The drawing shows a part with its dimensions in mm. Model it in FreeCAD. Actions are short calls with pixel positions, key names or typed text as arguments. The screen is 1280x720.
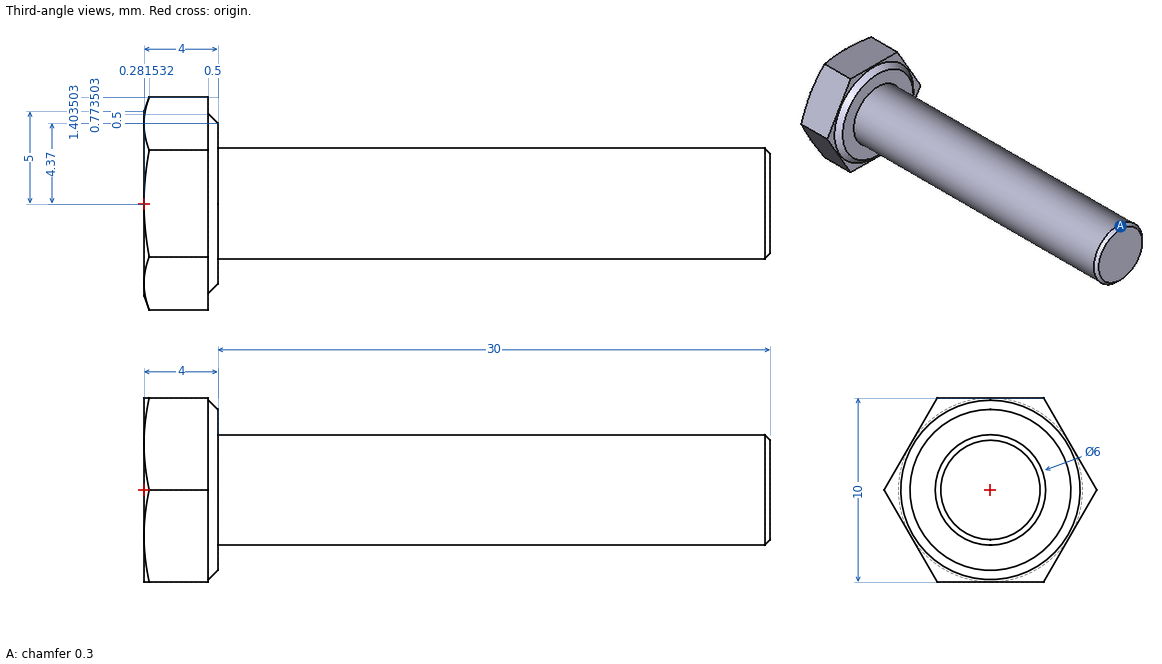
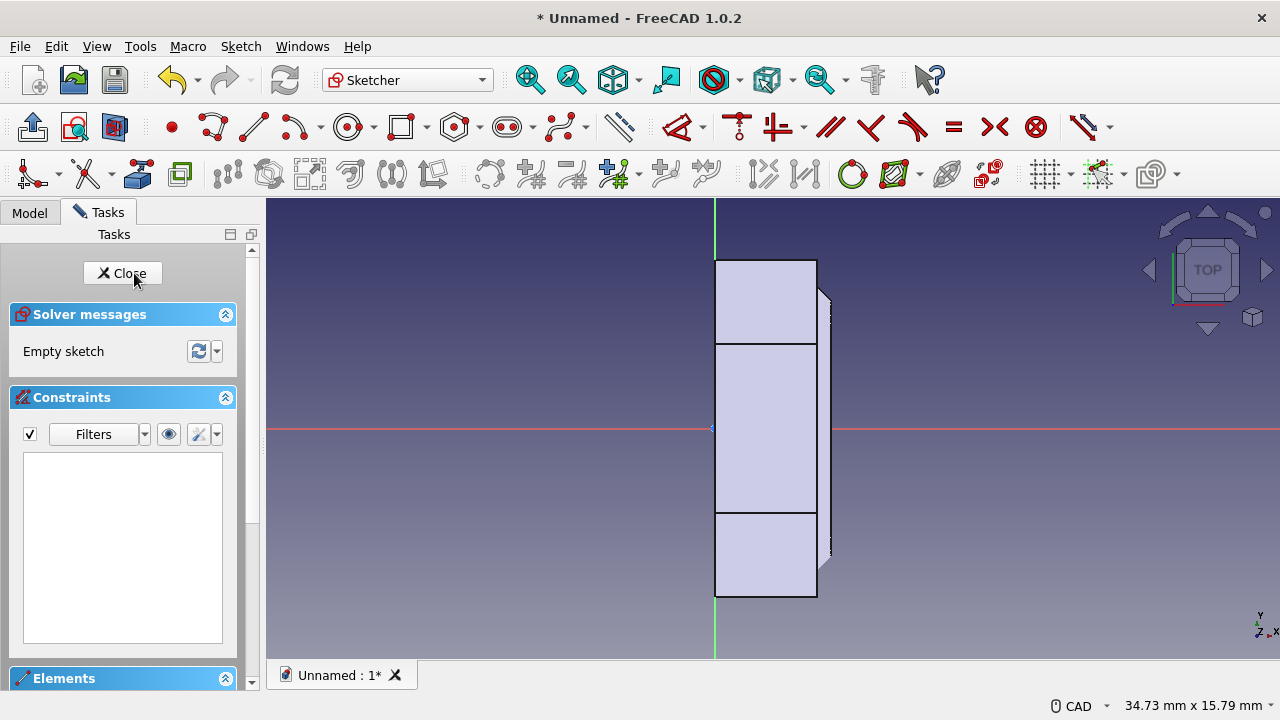
click(115, 128)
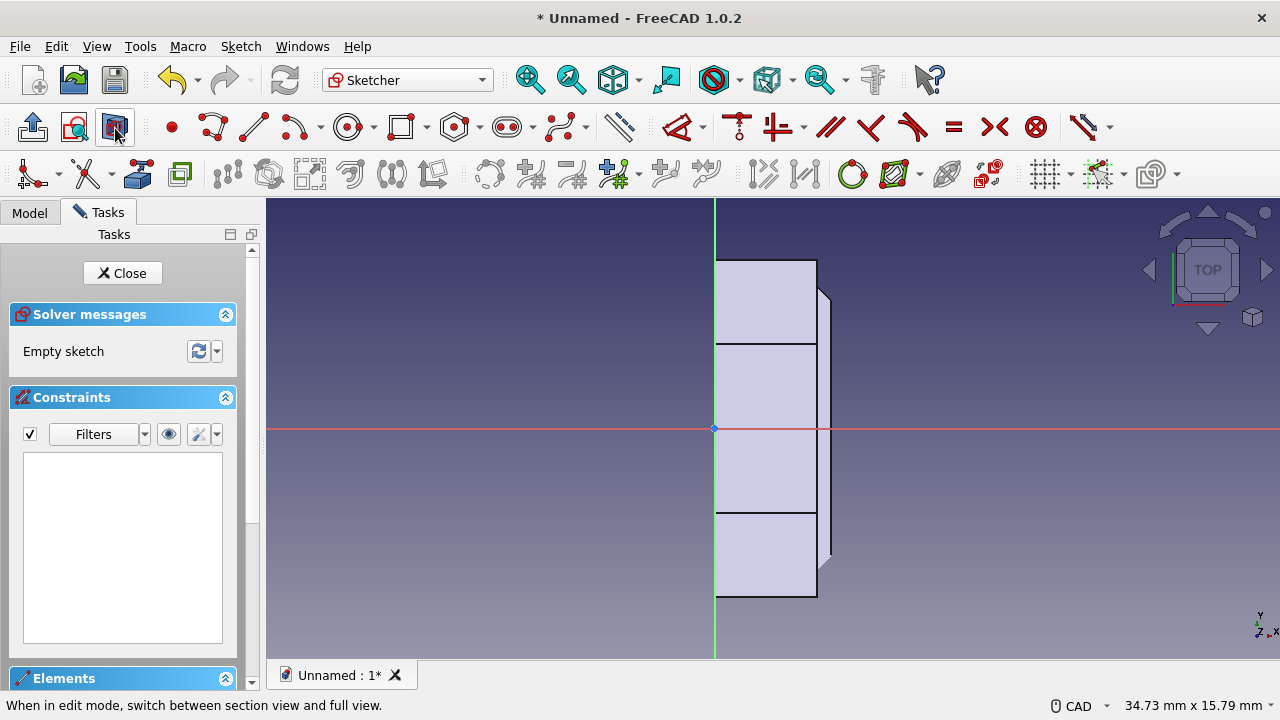
scroll(720, 259, up, 13)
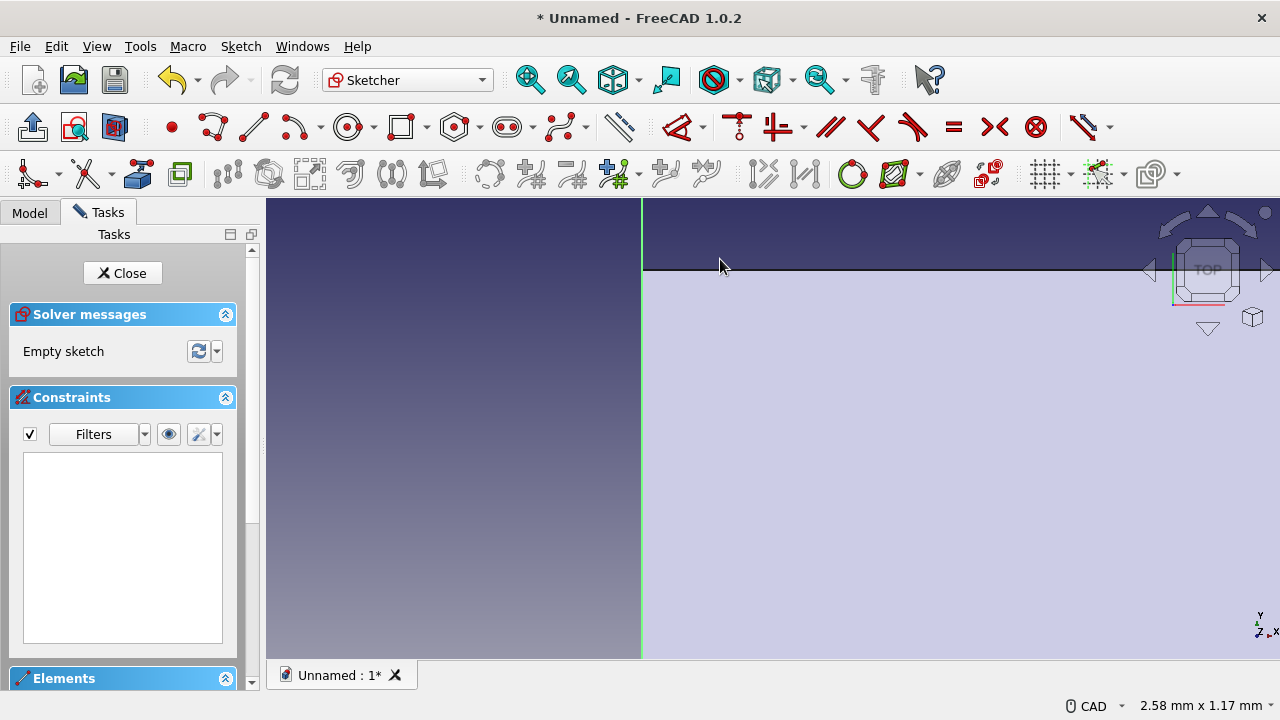
click(213, 128)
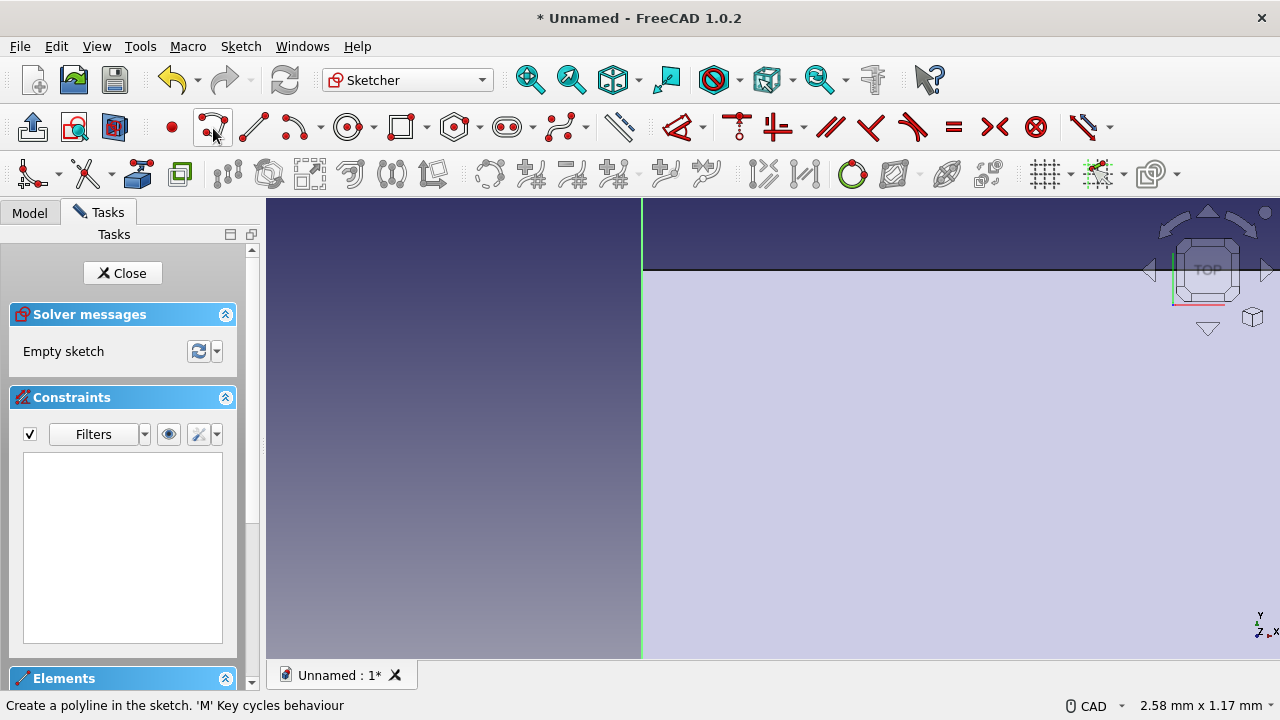
click(642, 574)
click(753, 270)
click(651, 270)
click(642, 575)
key(Escape)
key(Escape)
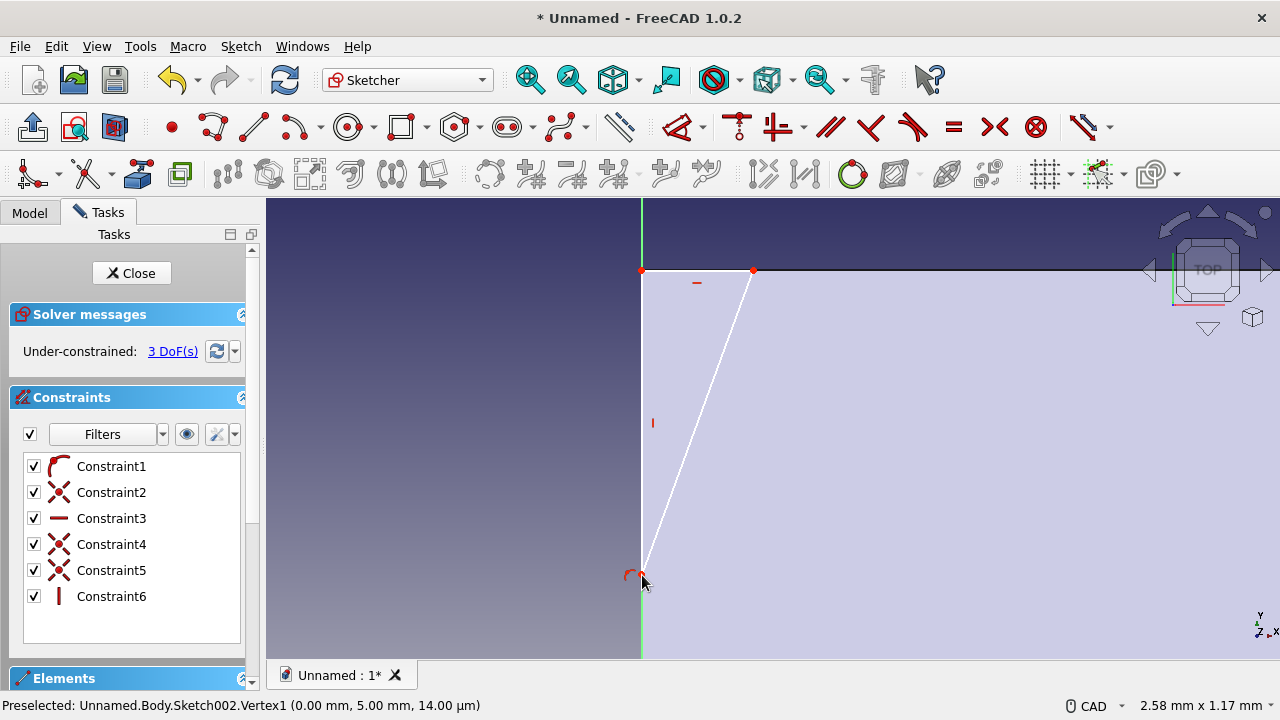
click(676, 128)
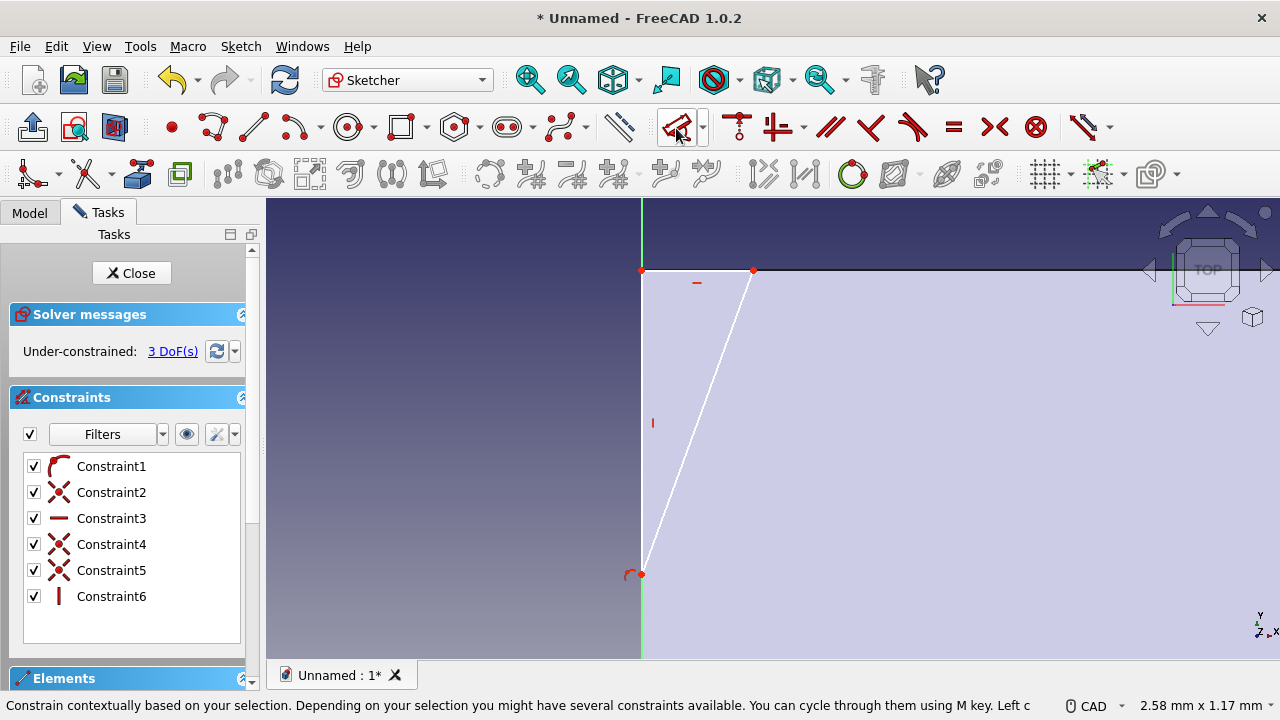
click(642, 575)
click(608, 603)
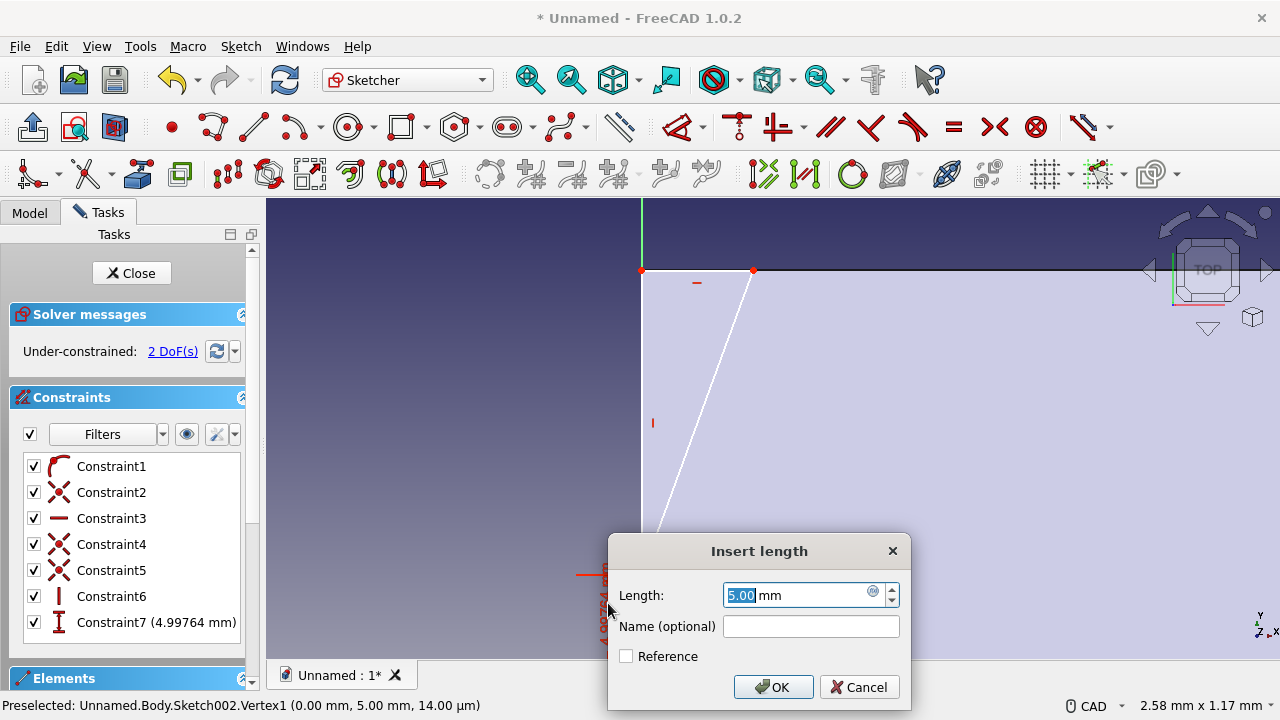
text(5)
key(Return)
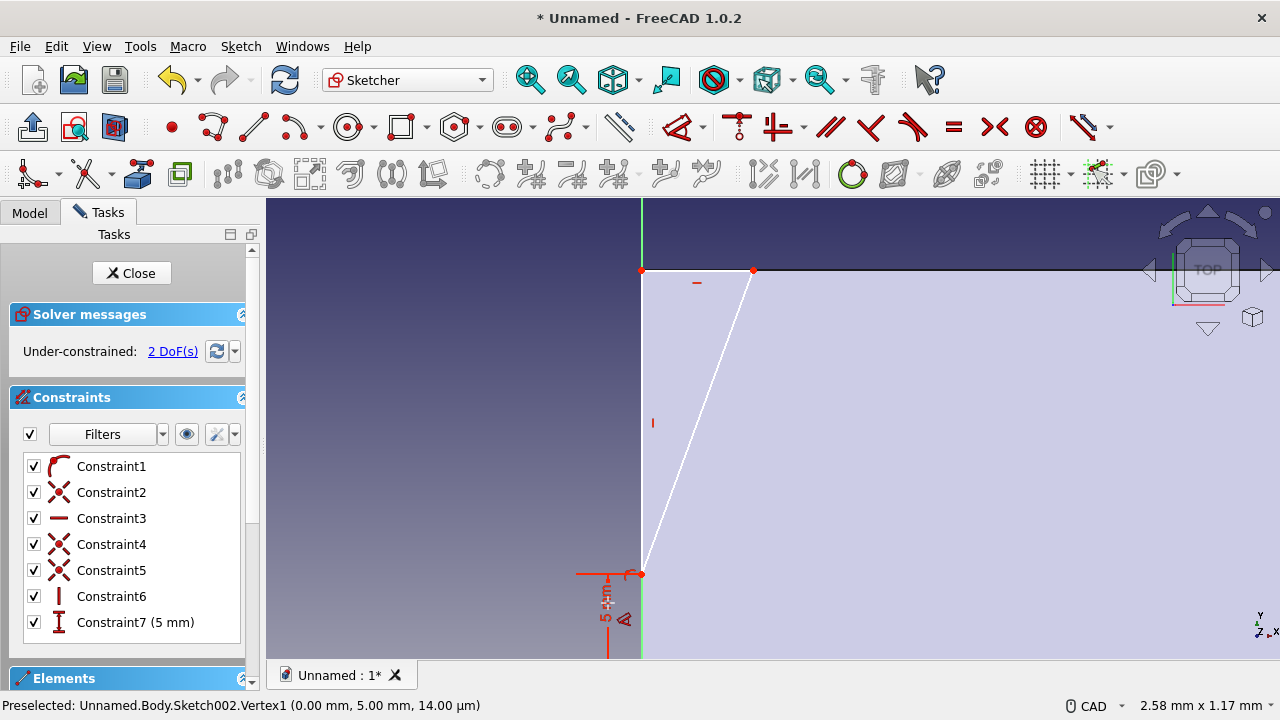
click(720, 271)
click(697, 237)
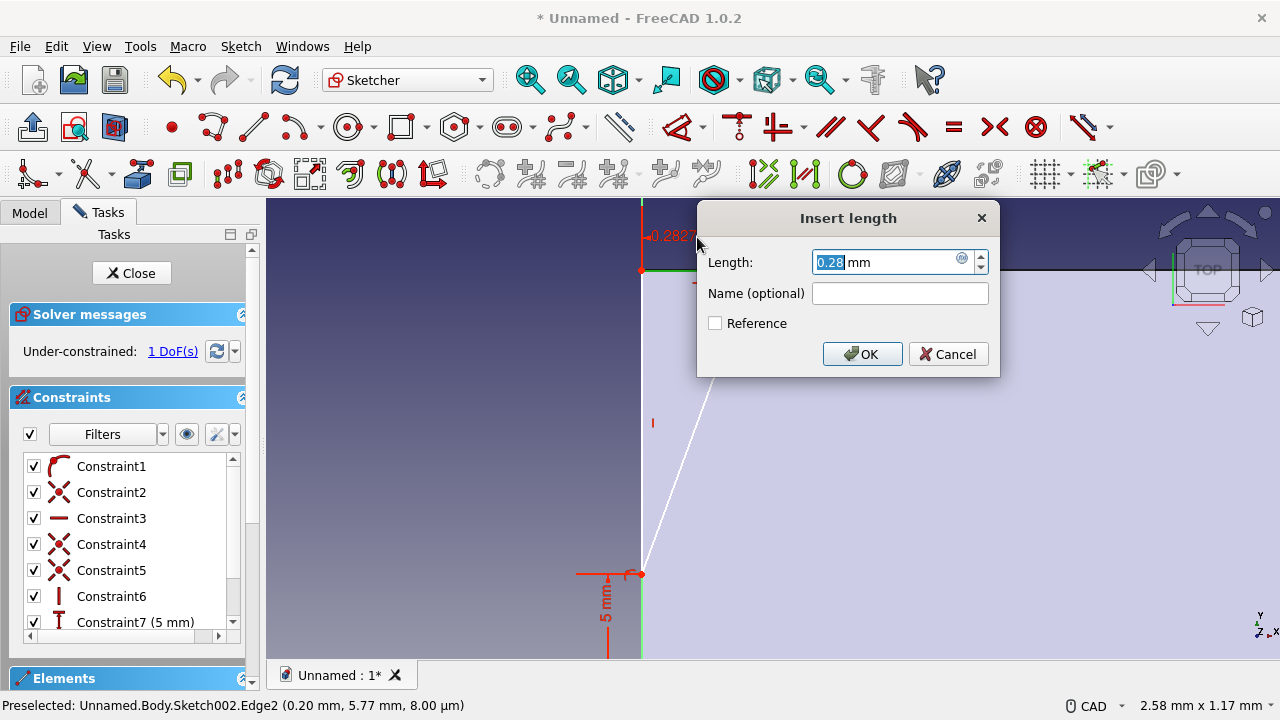
text(0.281532)
key(Return)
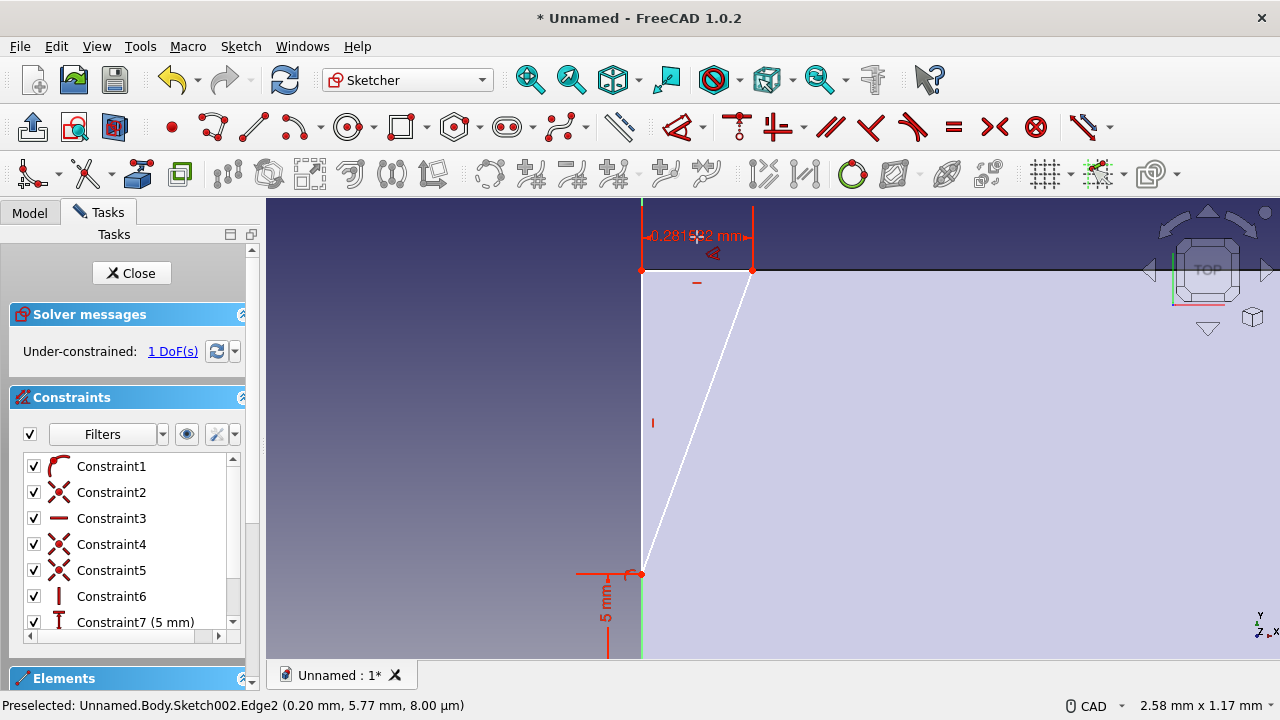
click(642, 362)
click(608, 423)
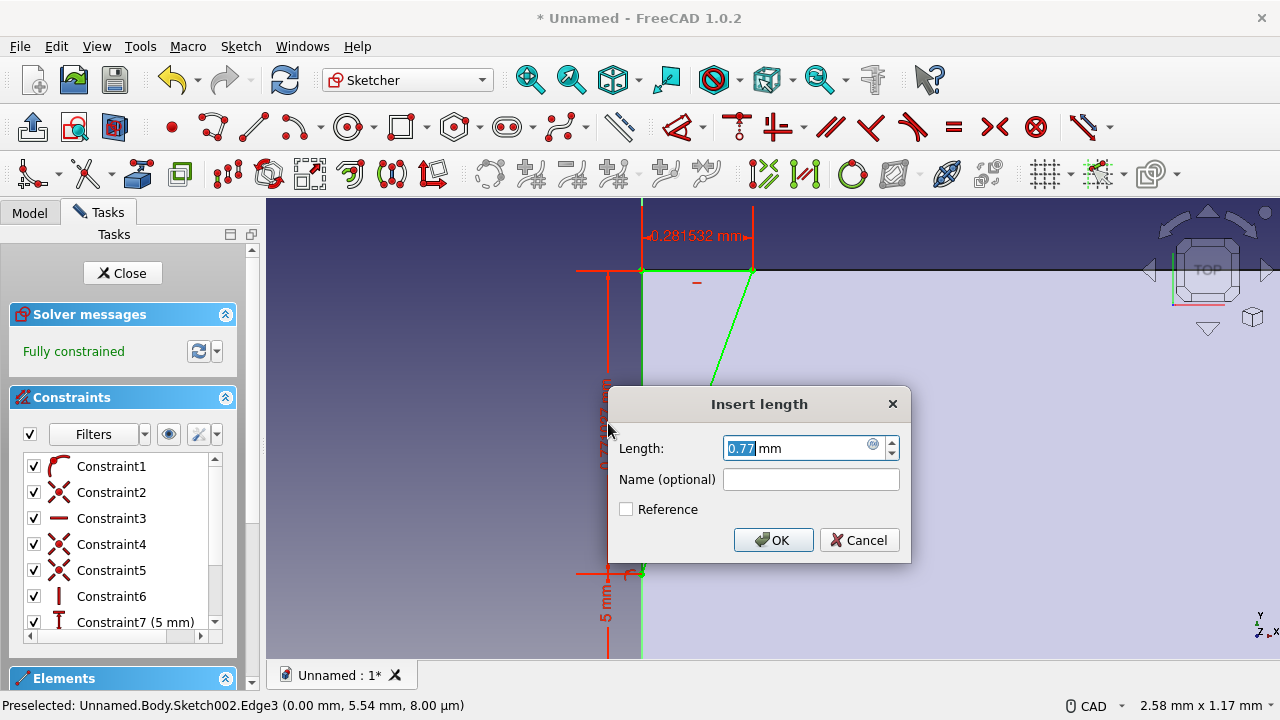
text(0.773503)
key(Return)
key(Escape)